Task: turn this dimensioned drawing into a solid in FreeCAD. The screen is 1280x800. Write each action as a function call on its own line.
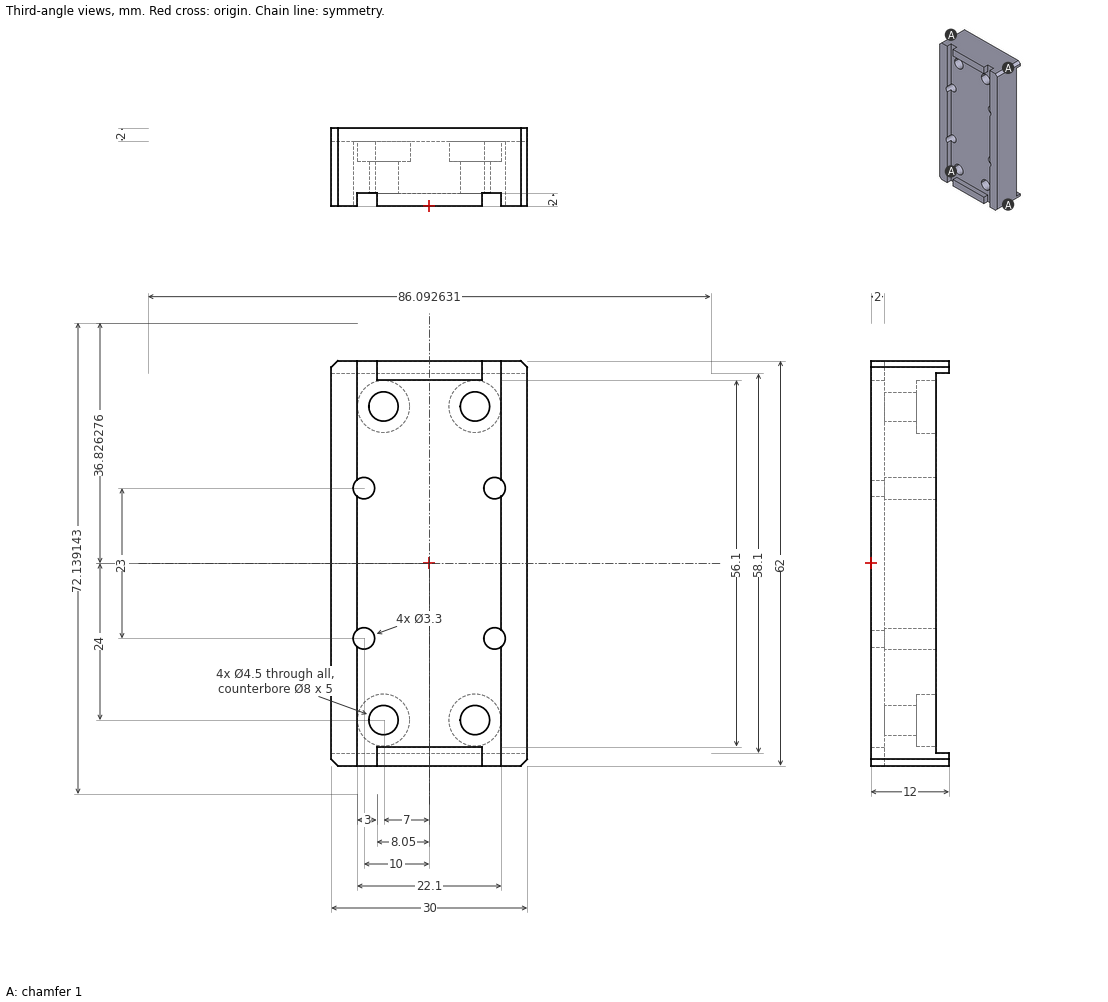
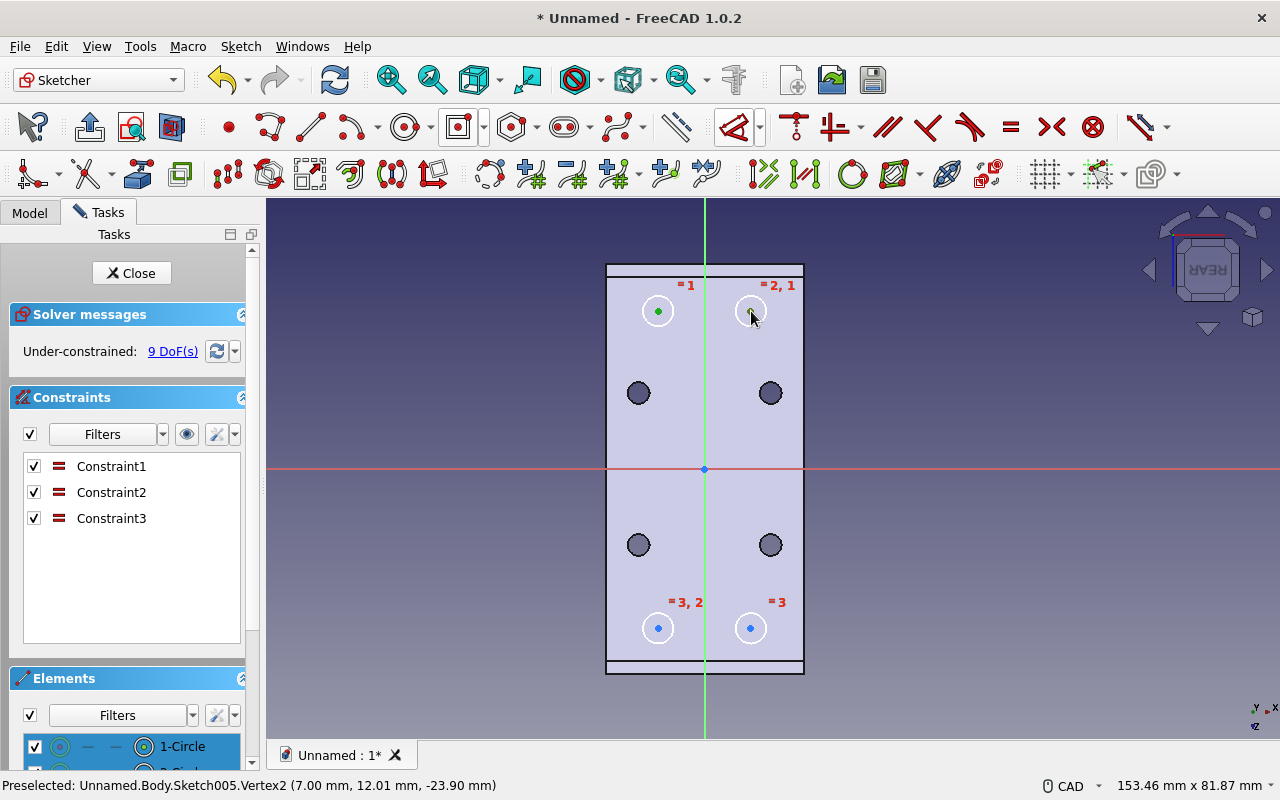
click(705, 676)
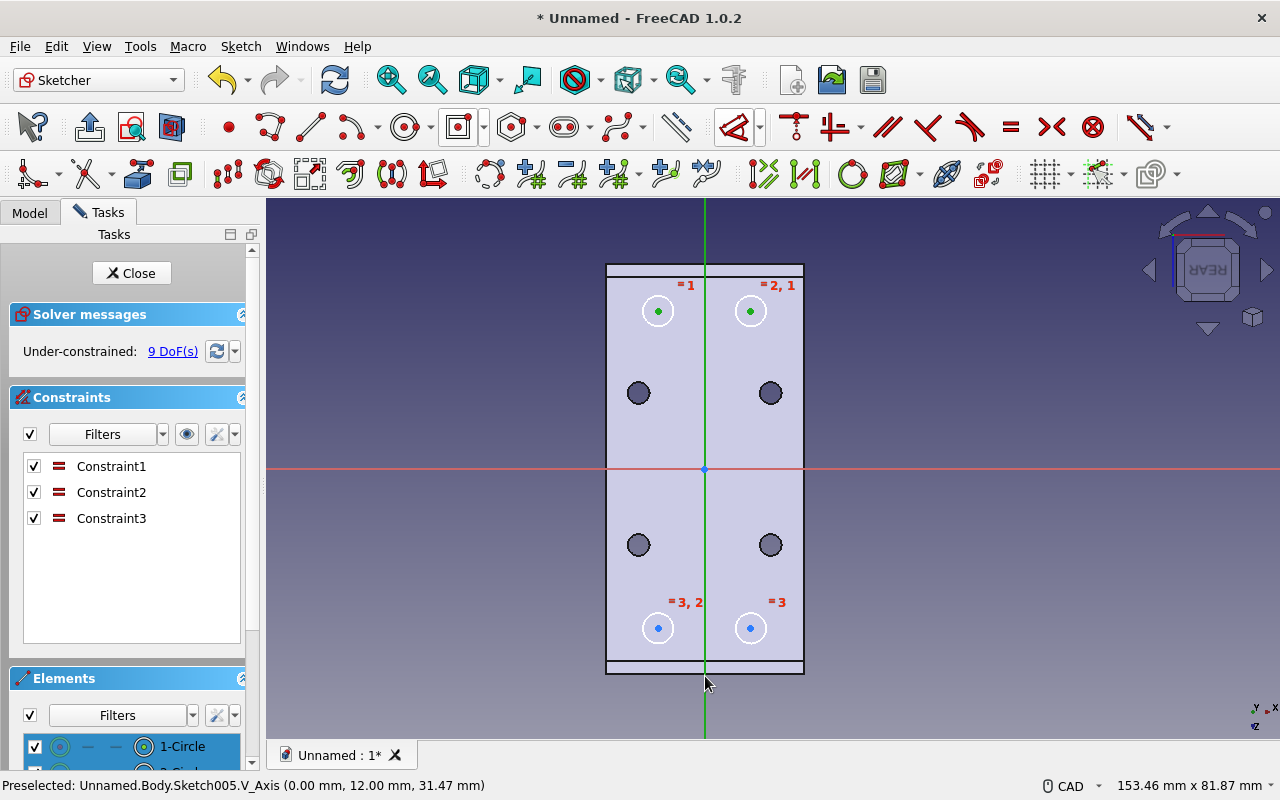
click(1052, 128)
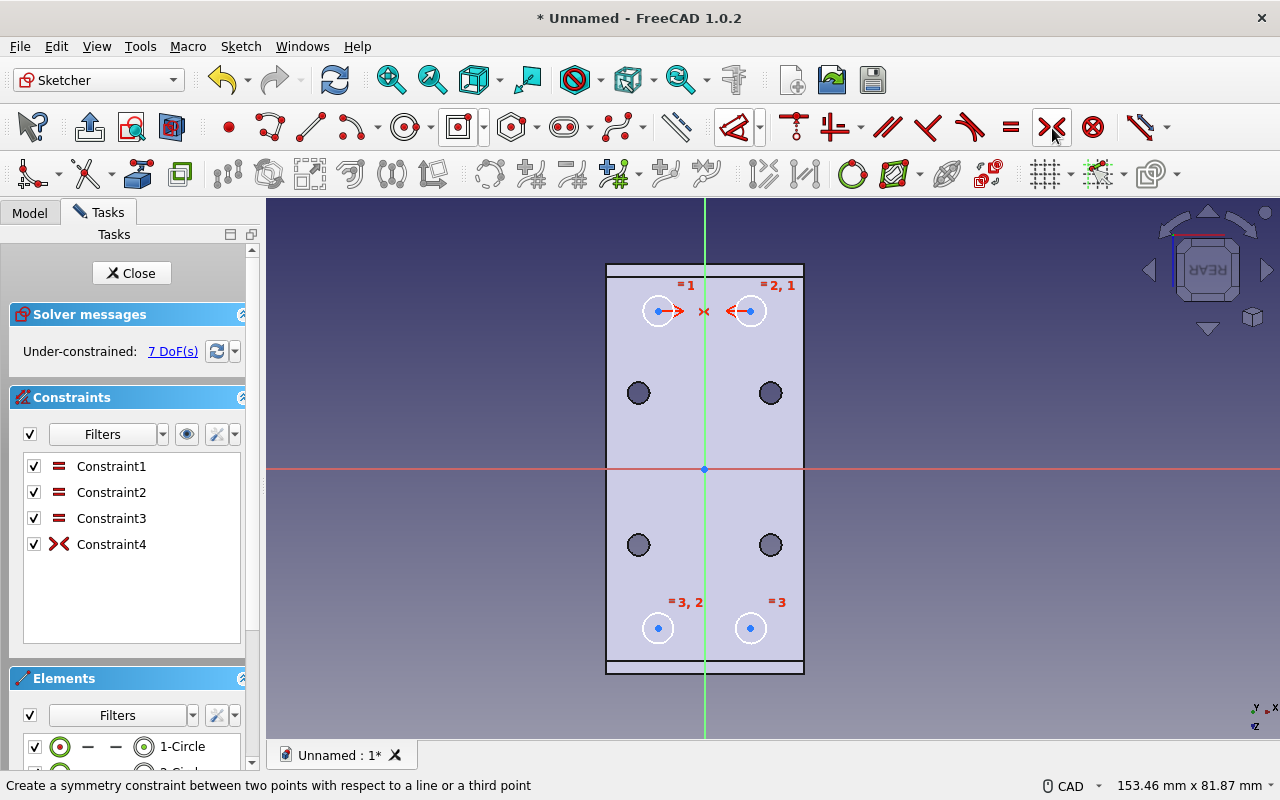
click(658, 311)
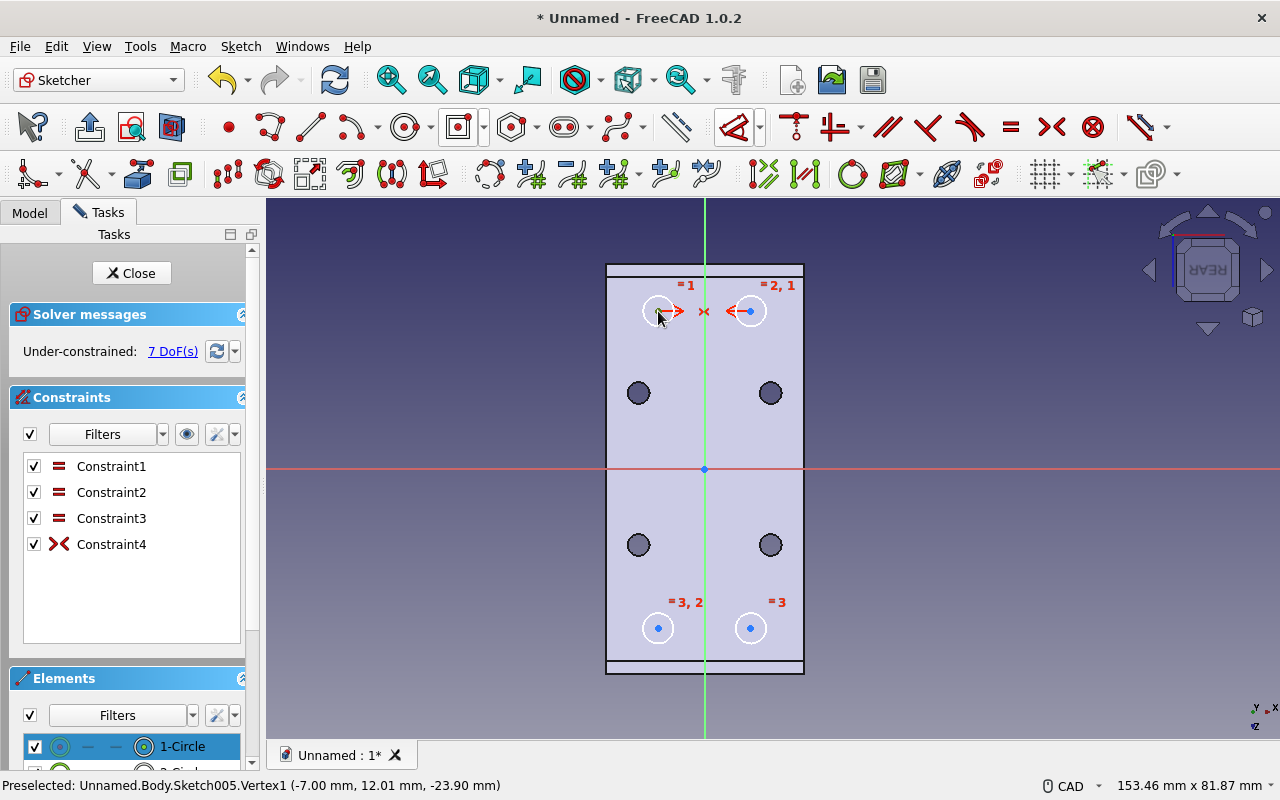
click(658, 628)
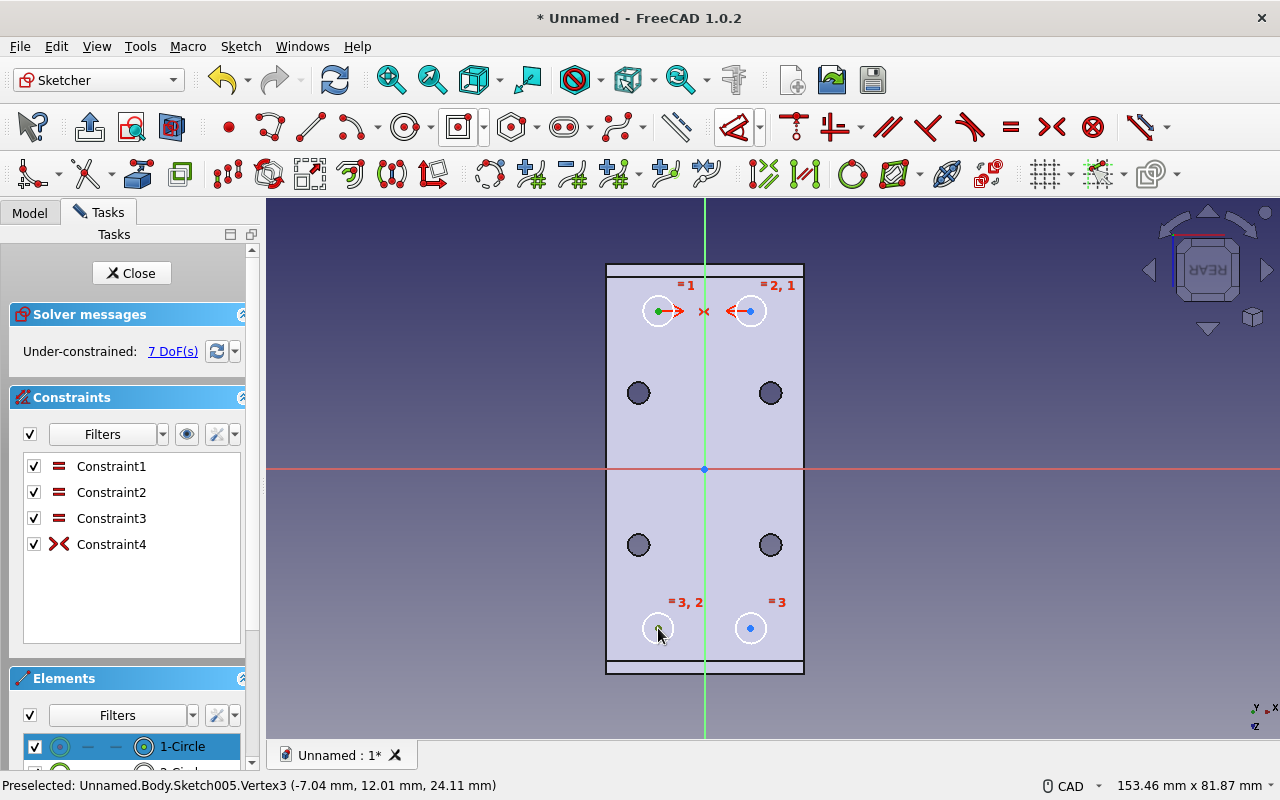
click(353, 469)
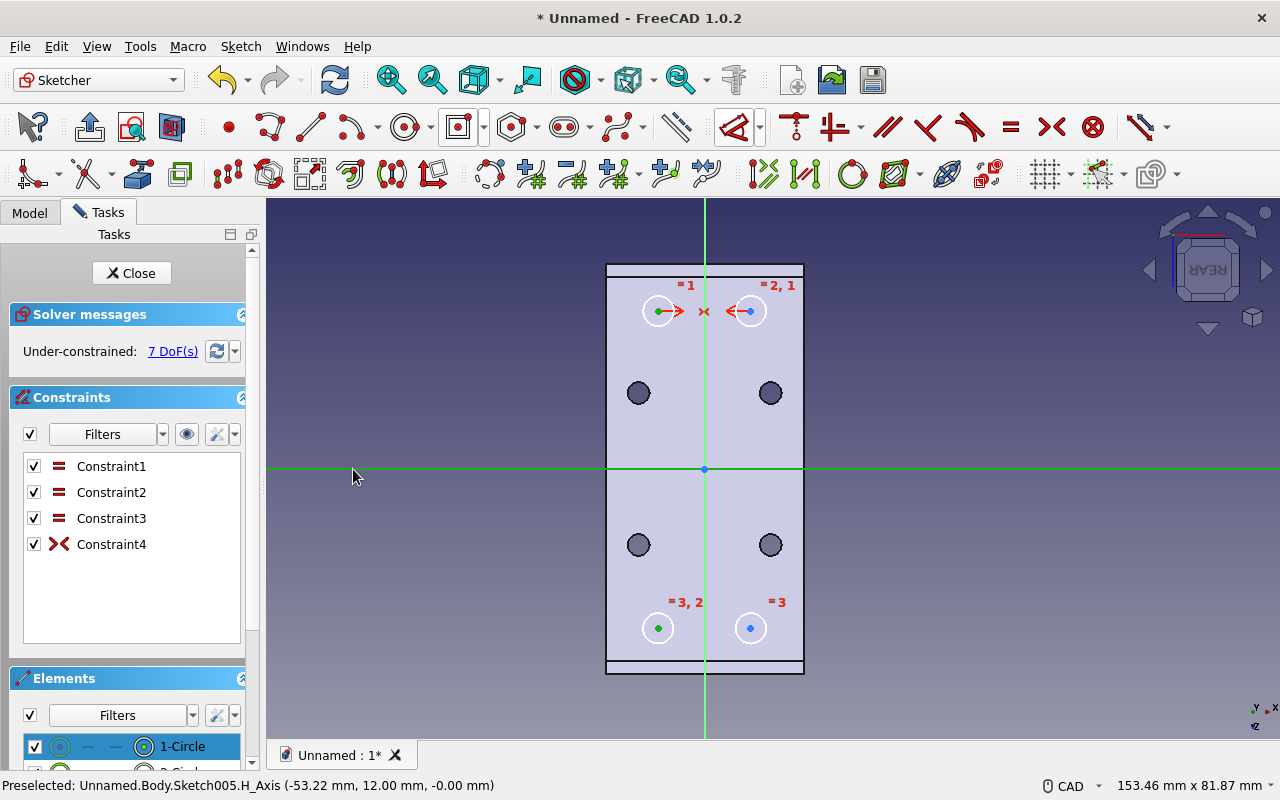
click(1052, 128)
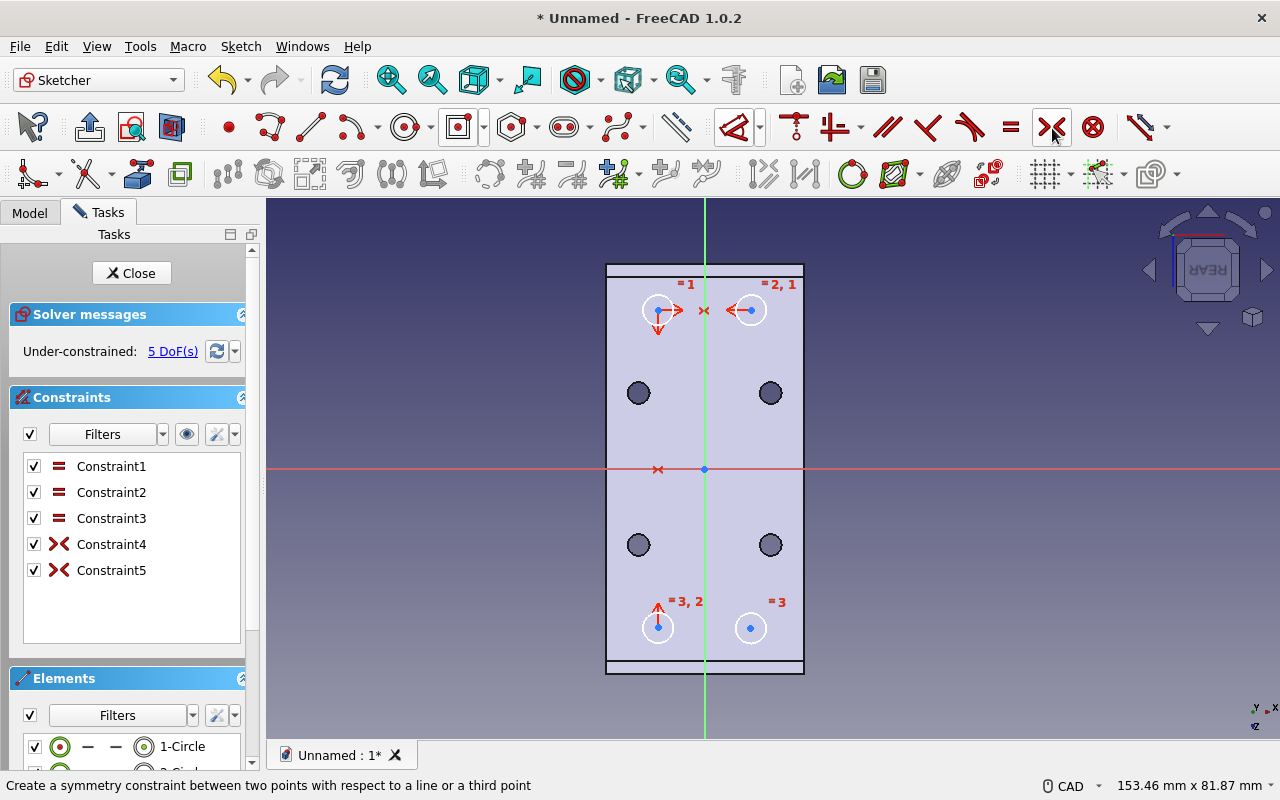
click(751, 310)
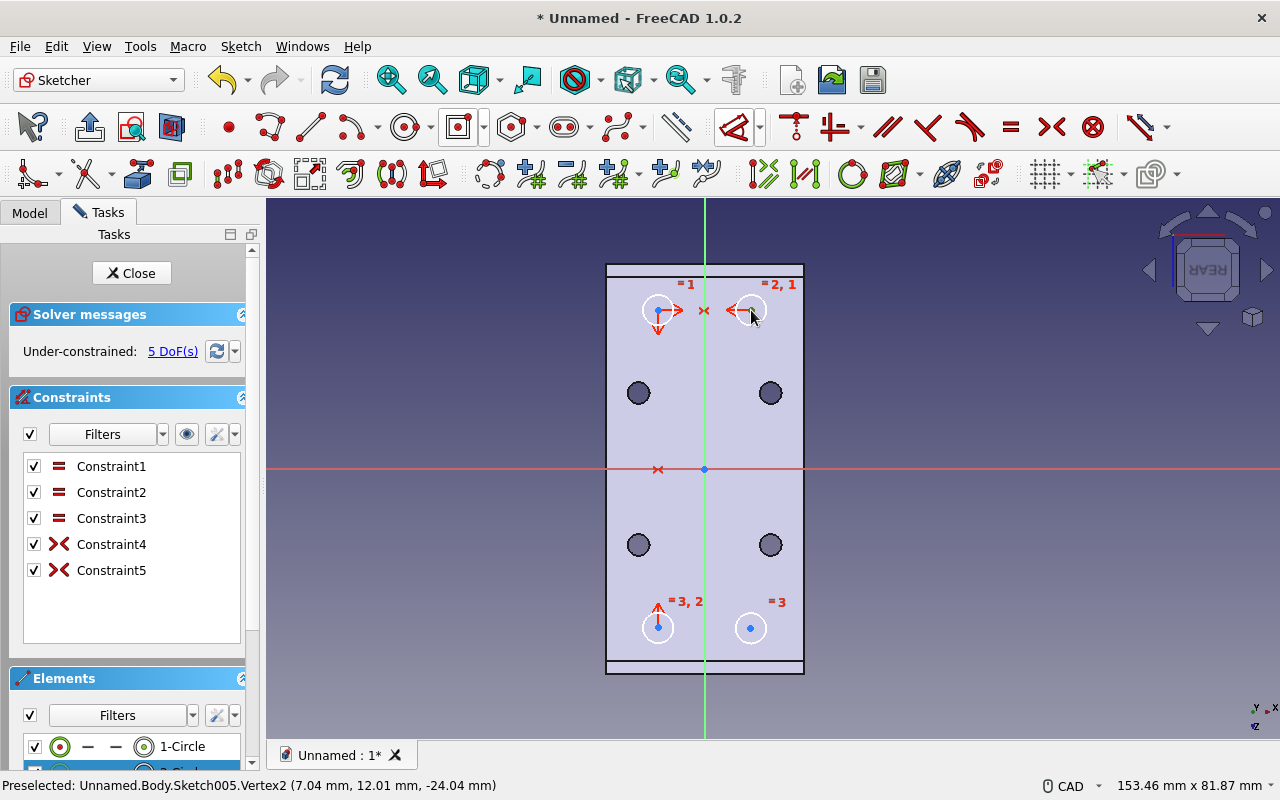
click(751, 628)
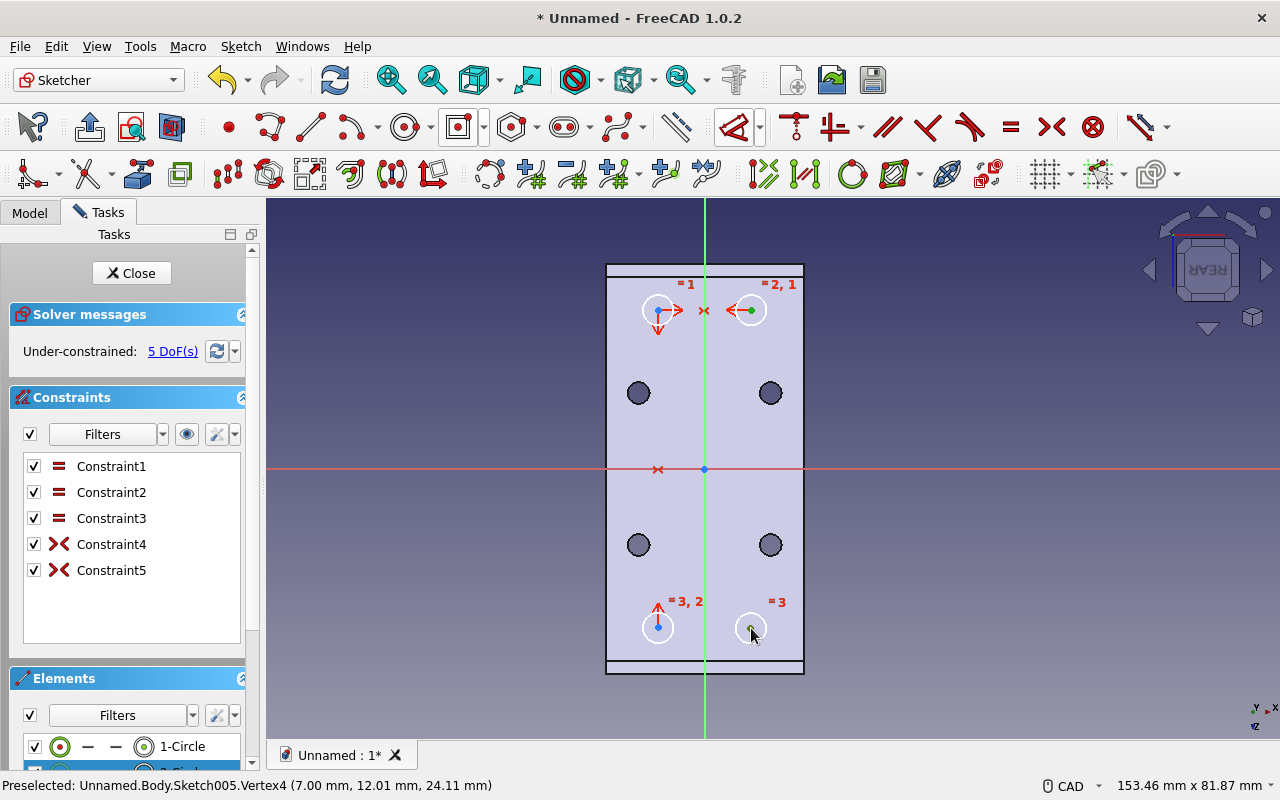
click(353, 469)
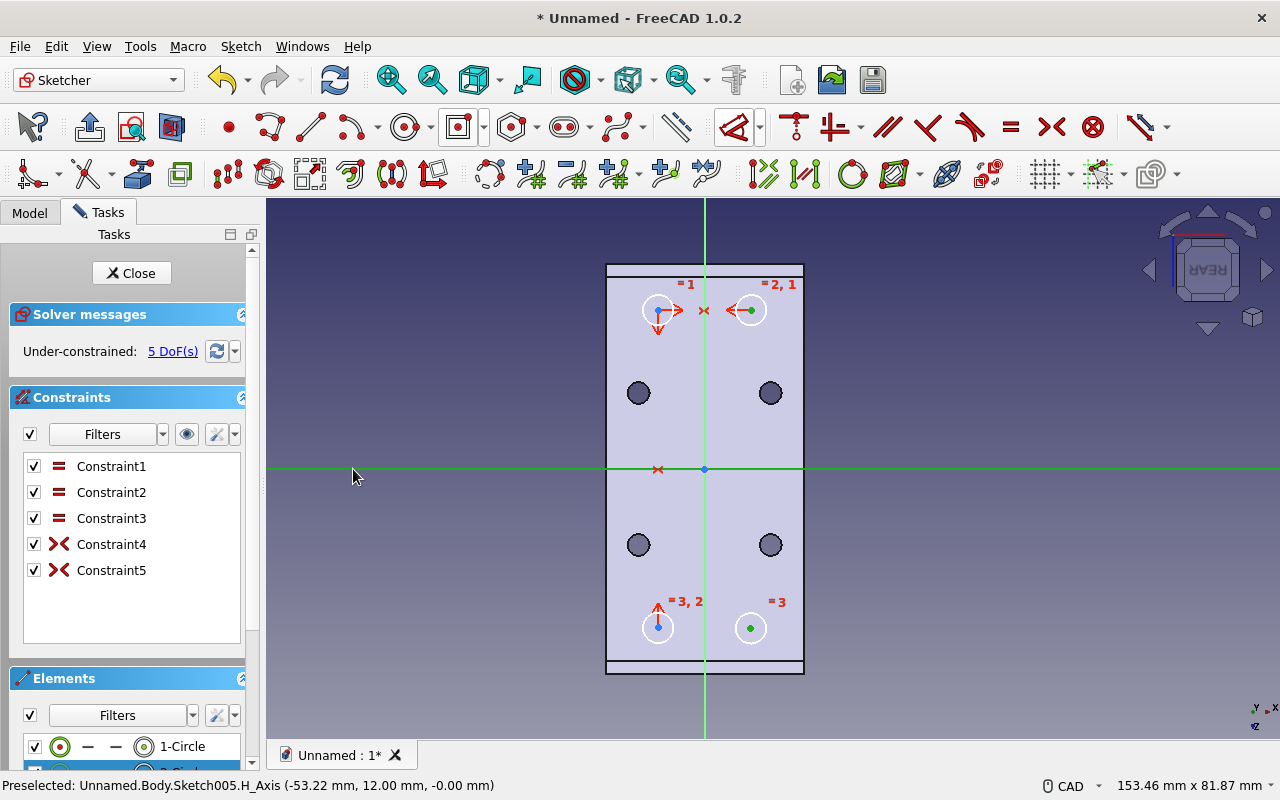
click(1052, 128)